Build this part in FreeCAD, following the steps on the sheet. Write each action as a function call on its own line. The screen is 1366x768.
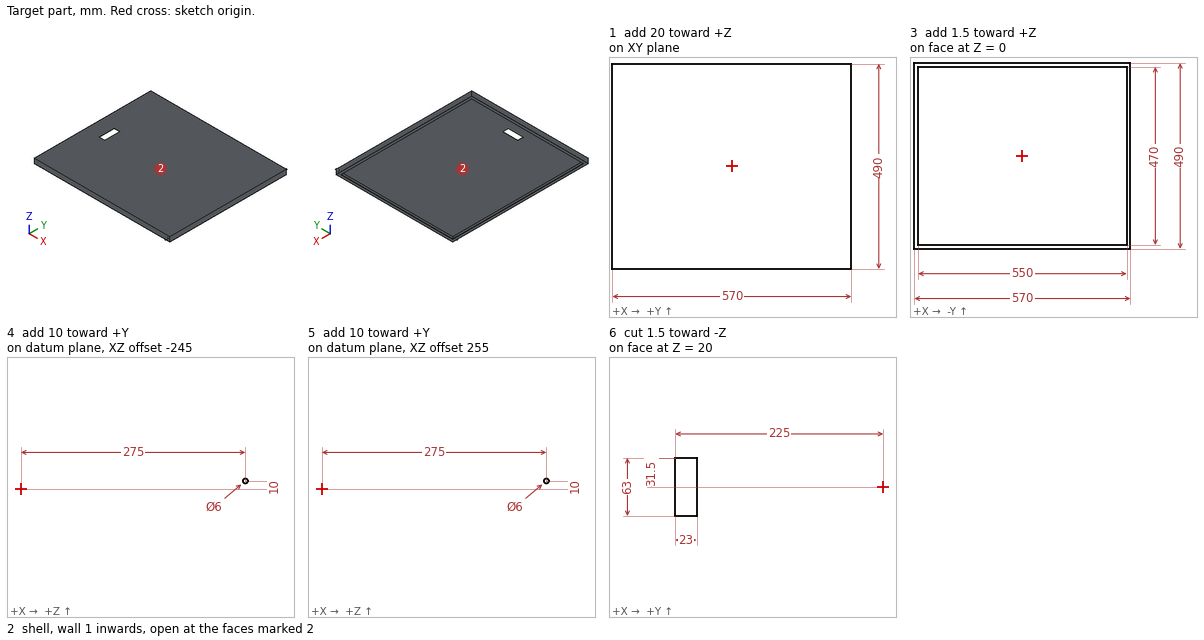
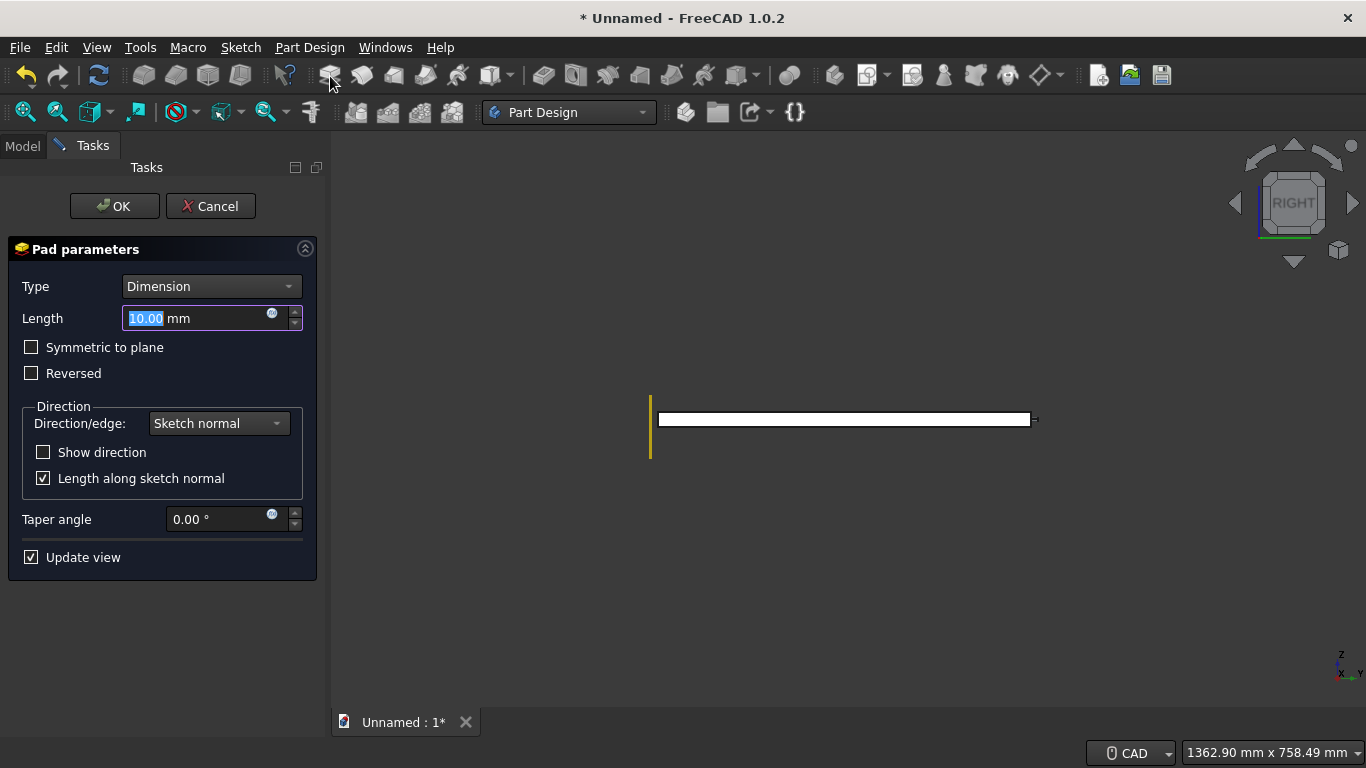
text(10)
key(Tab)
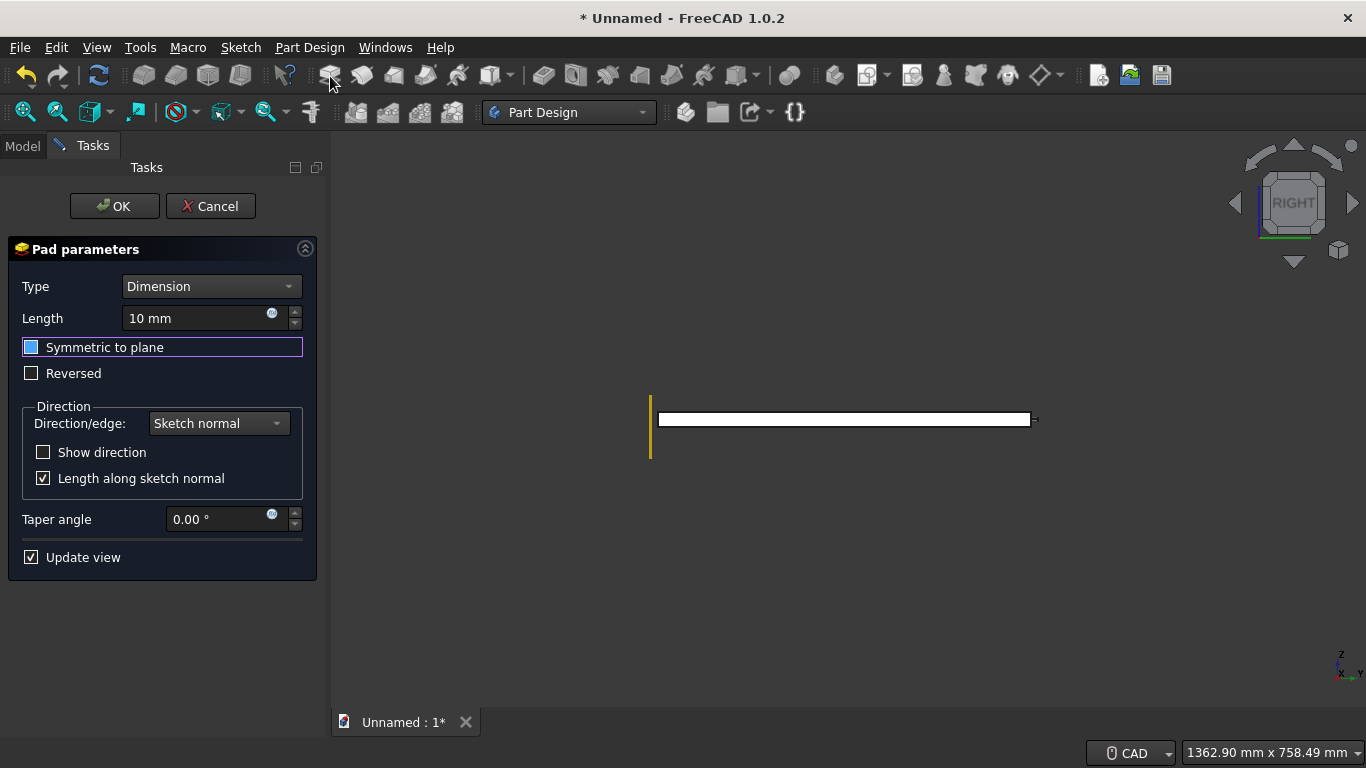
click(30, 373)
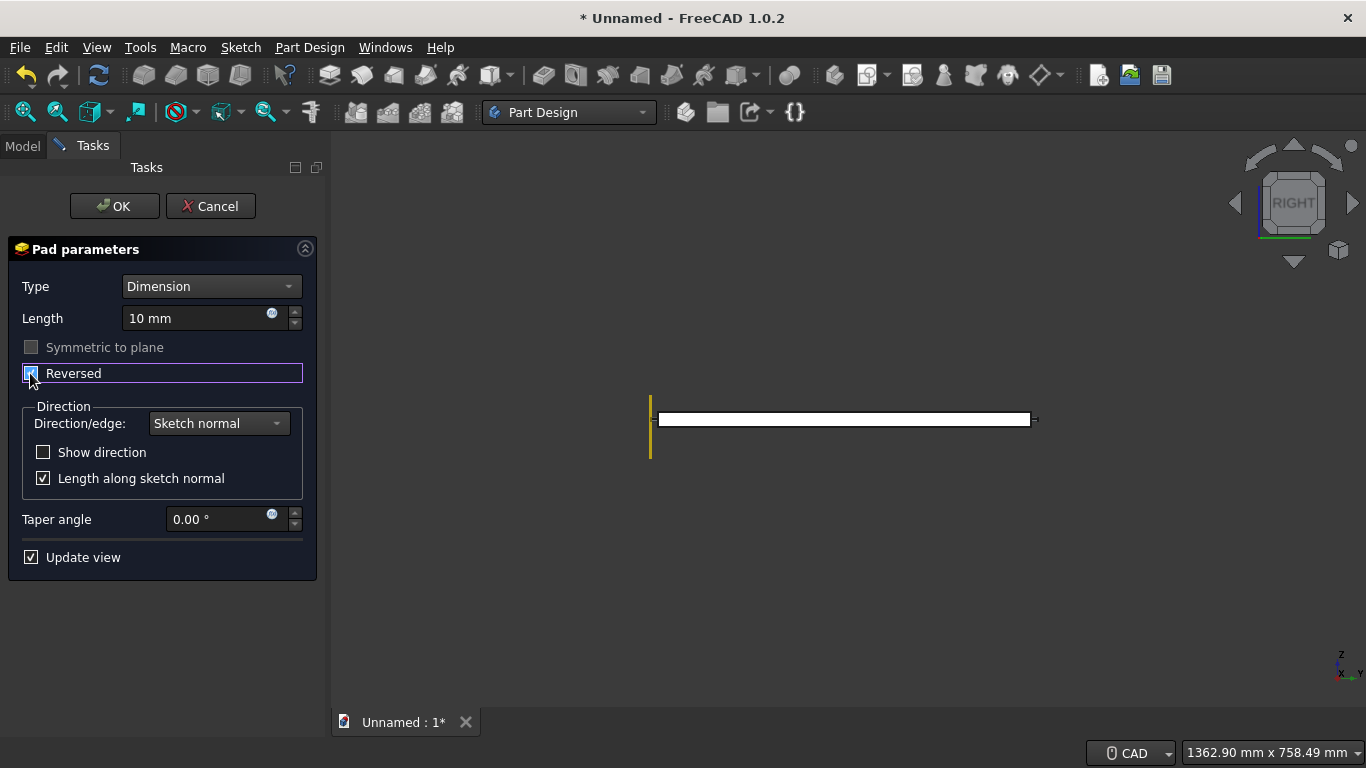
click(115, 206)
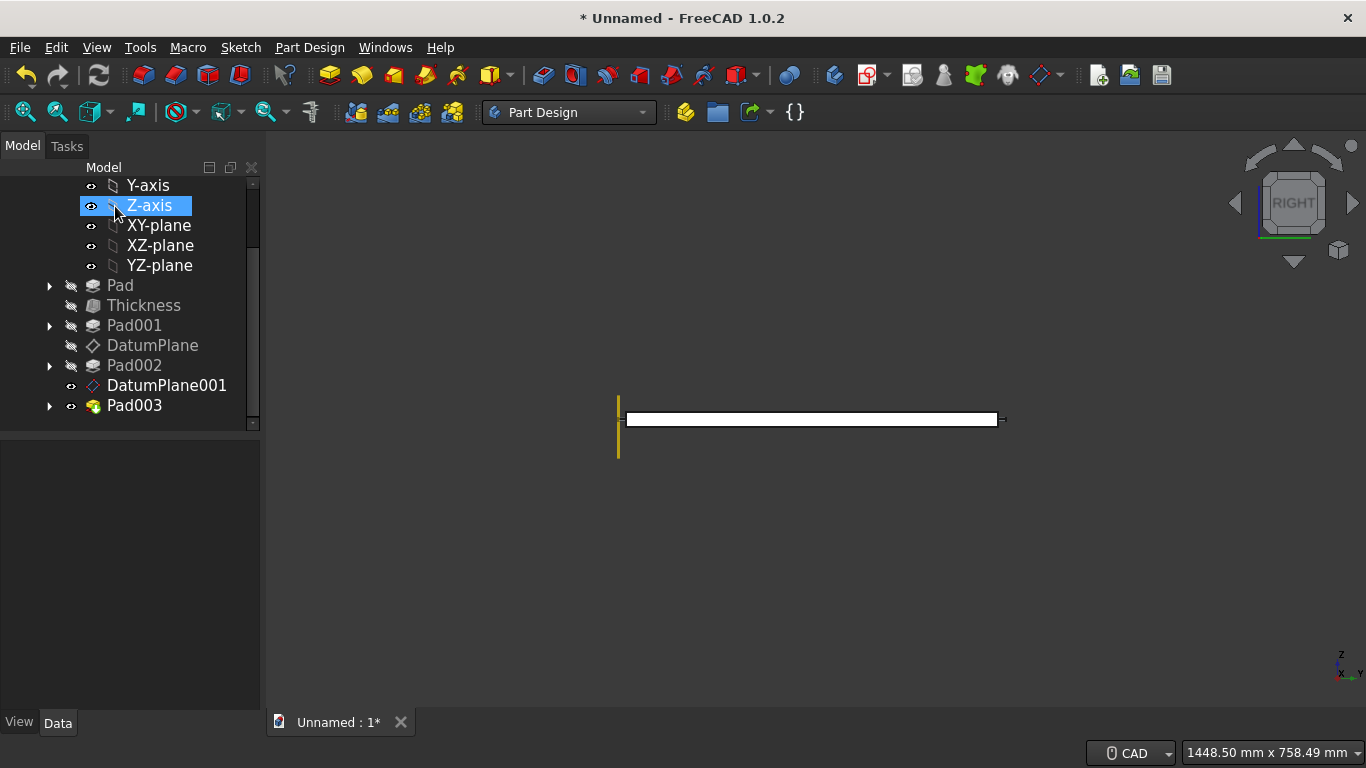
click(116, 386)
key(space)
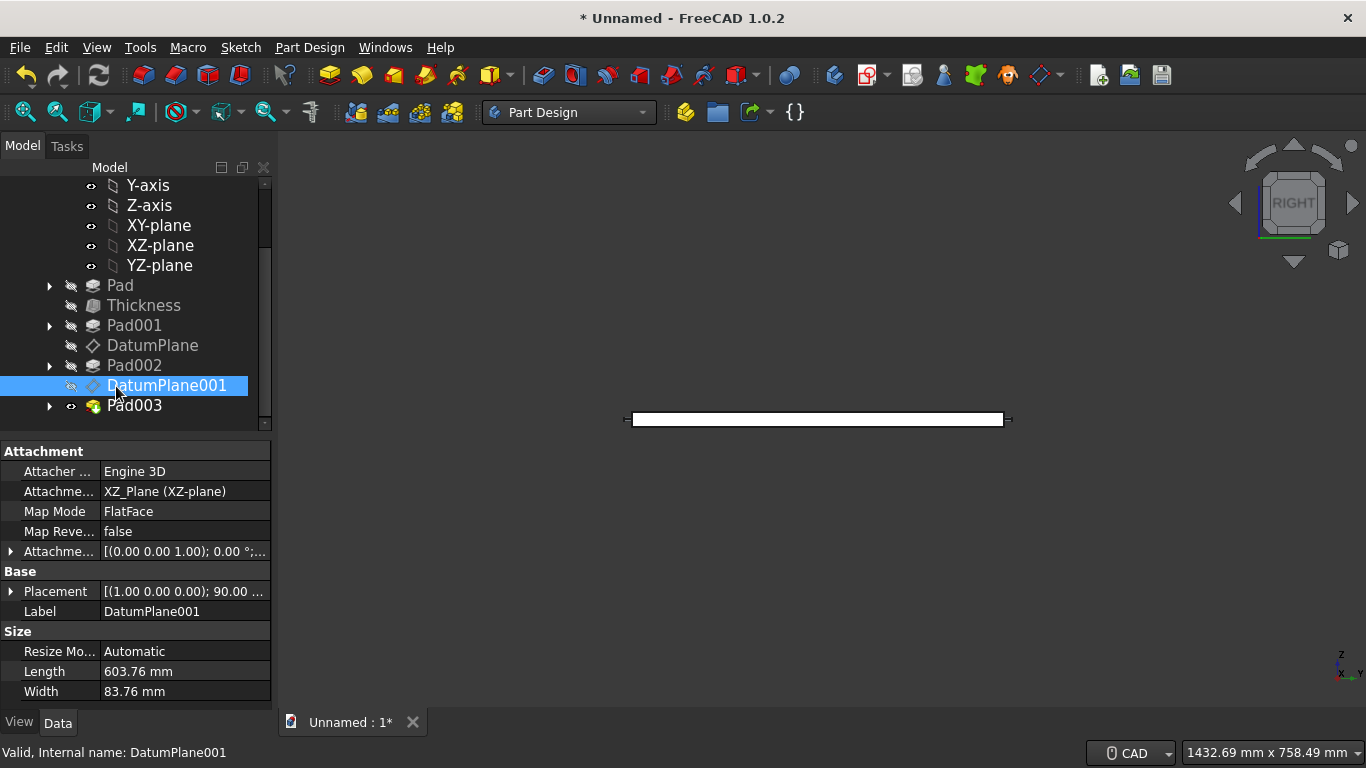
click(26, 112)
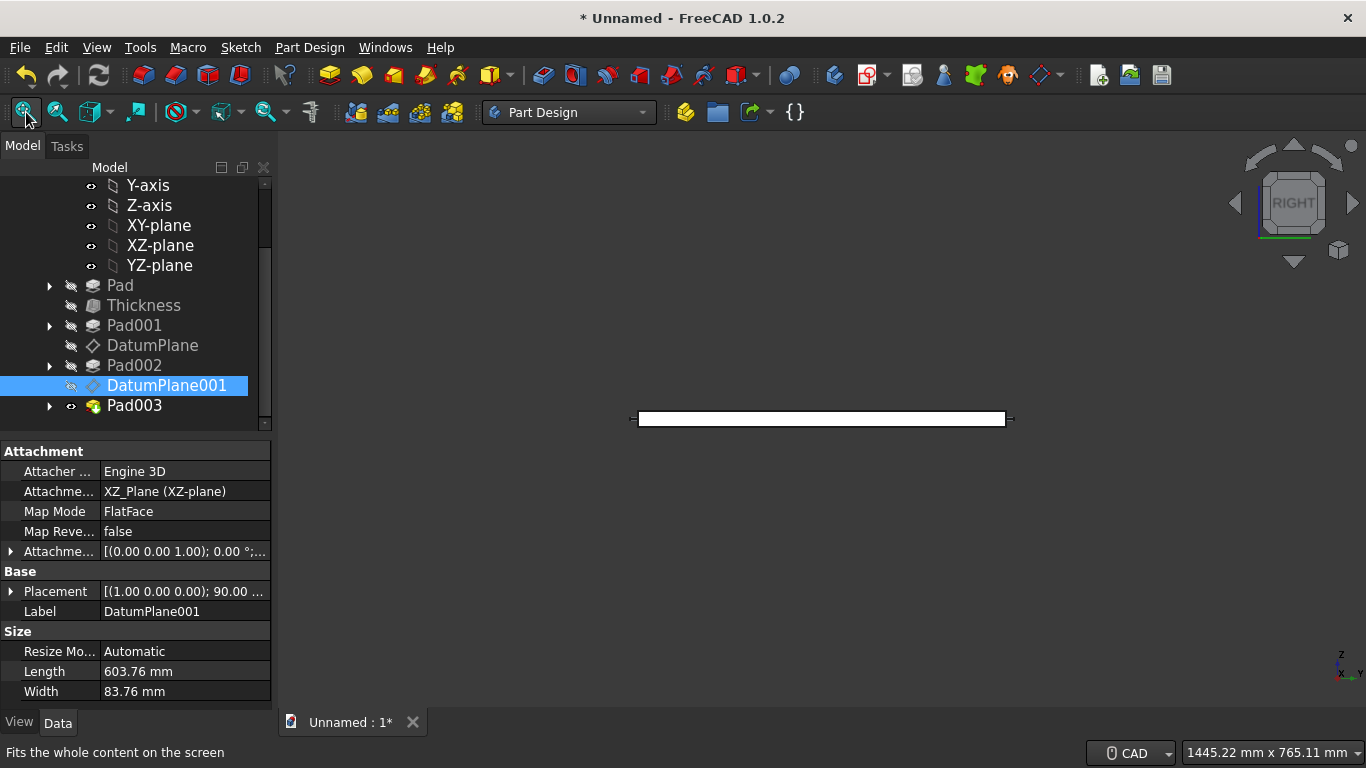
key(0)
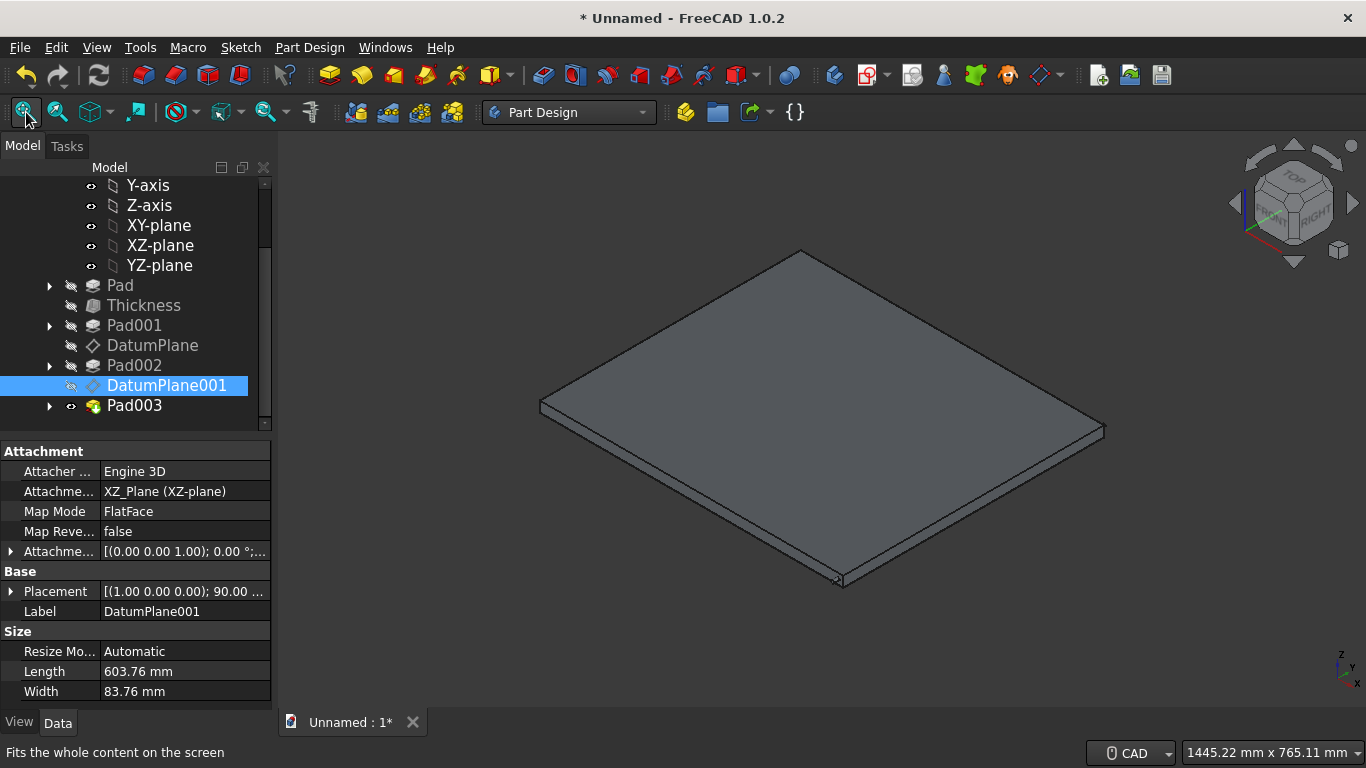
click(822, 412)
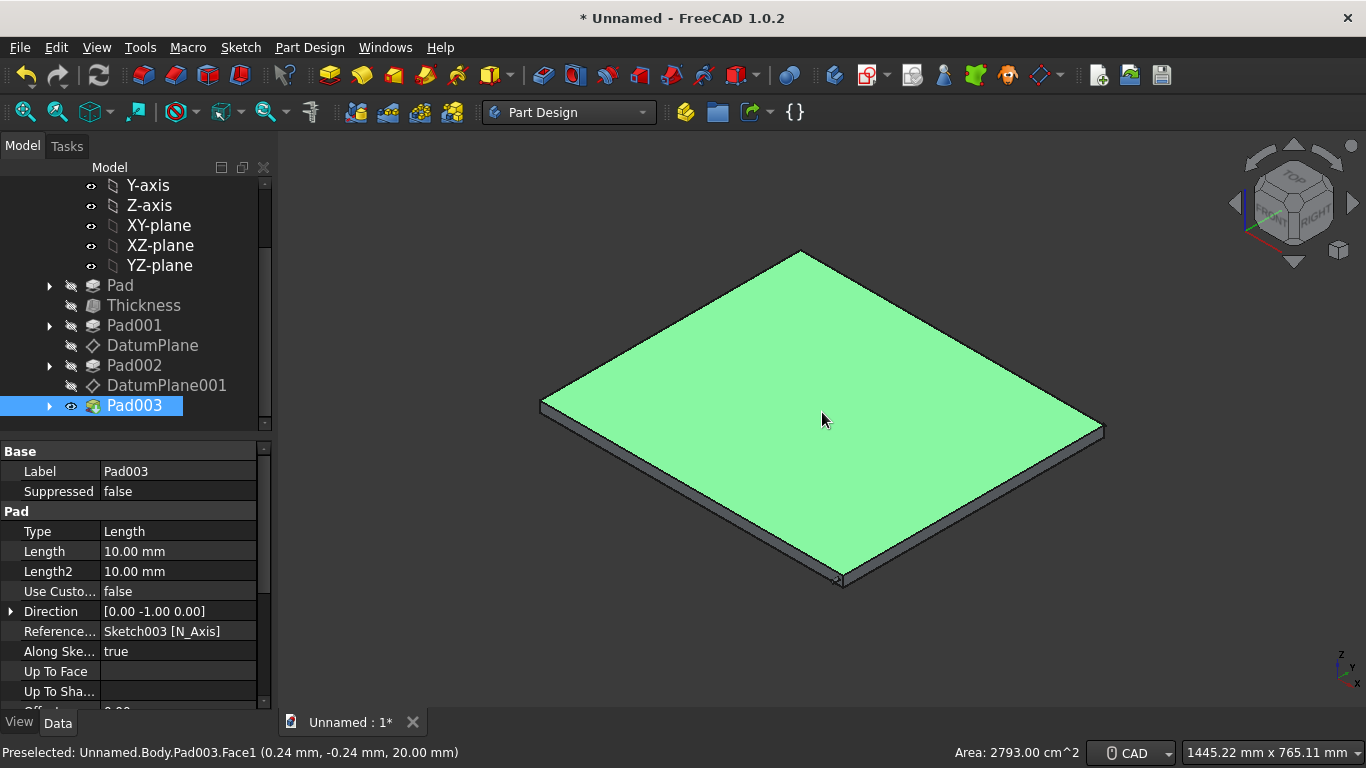
click(868, 76)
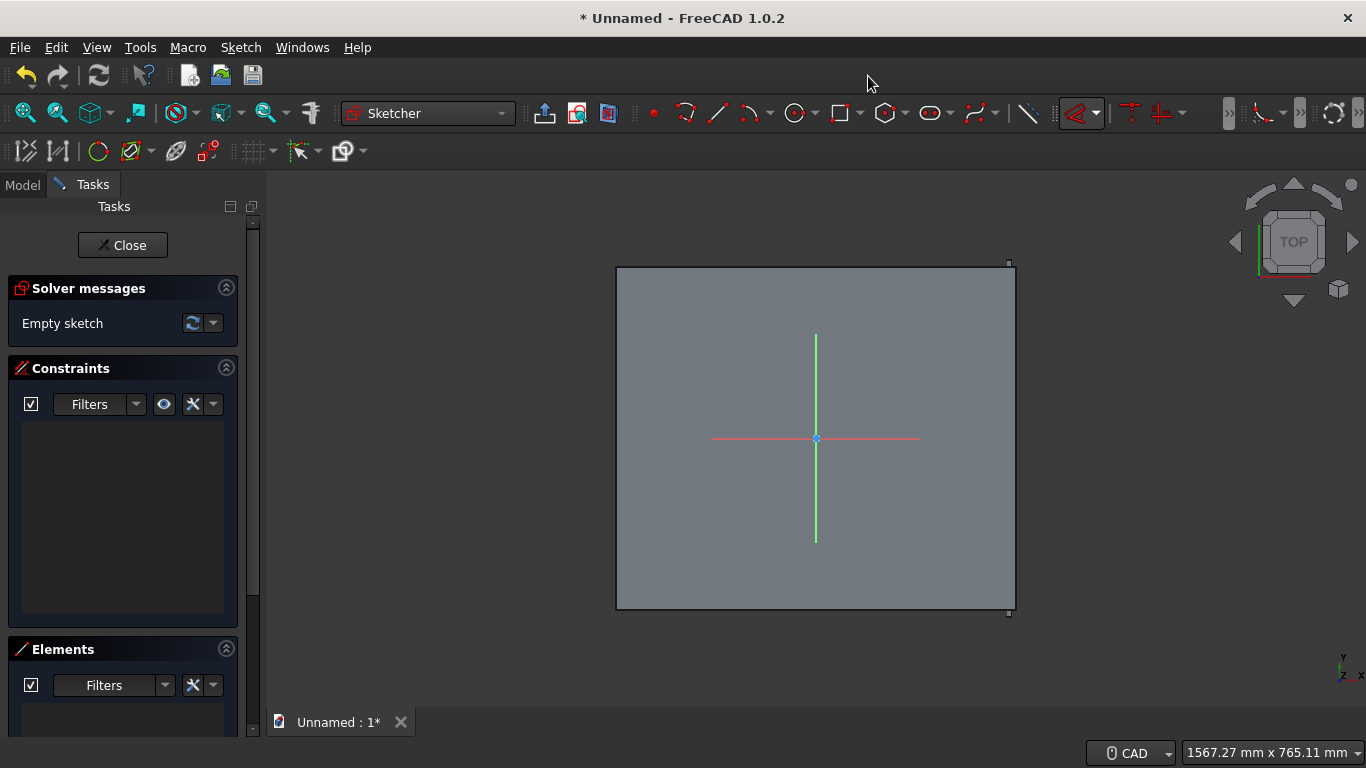
scroll(653, 439, up, 10)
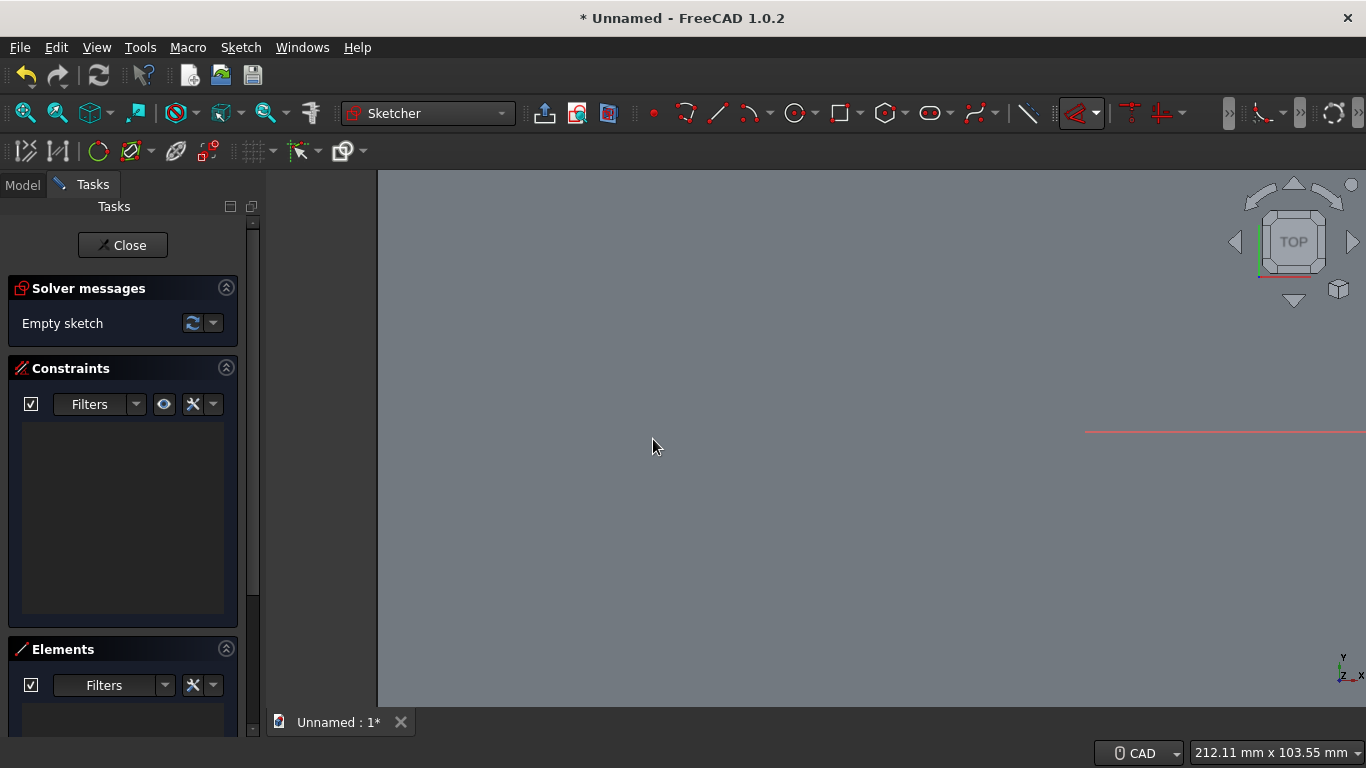
key(g)
key(r)